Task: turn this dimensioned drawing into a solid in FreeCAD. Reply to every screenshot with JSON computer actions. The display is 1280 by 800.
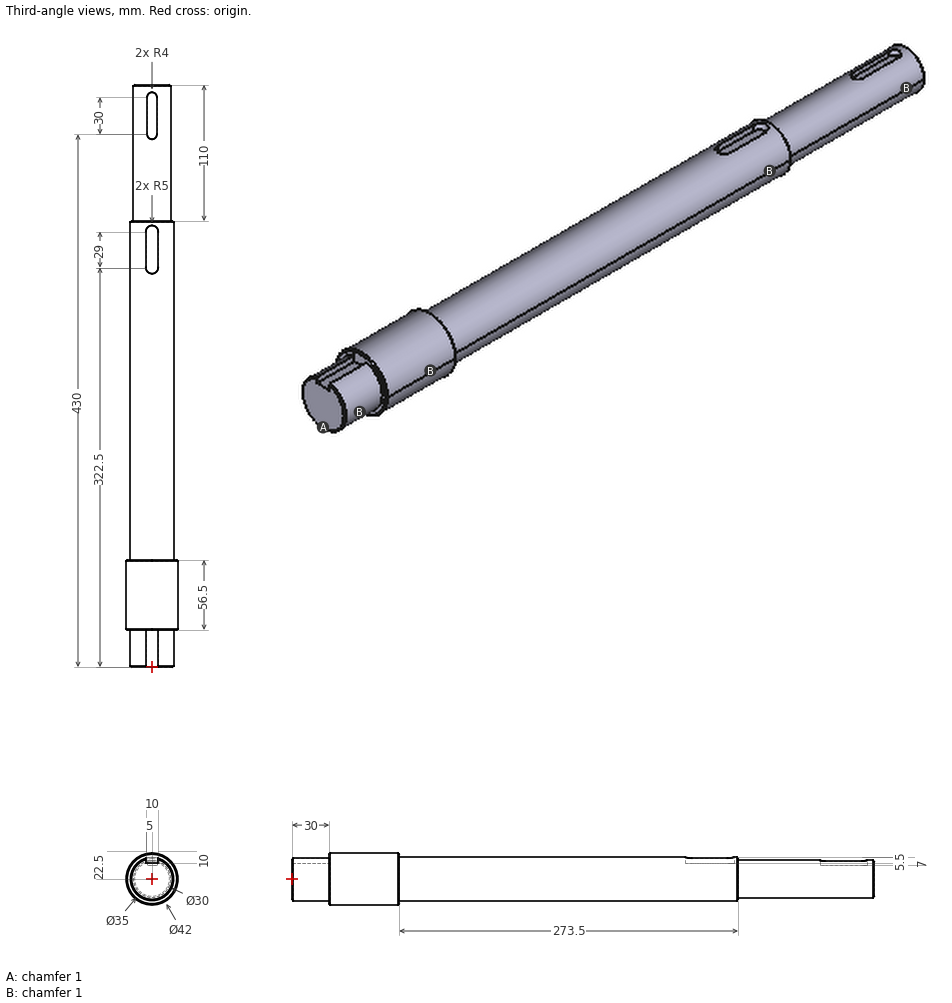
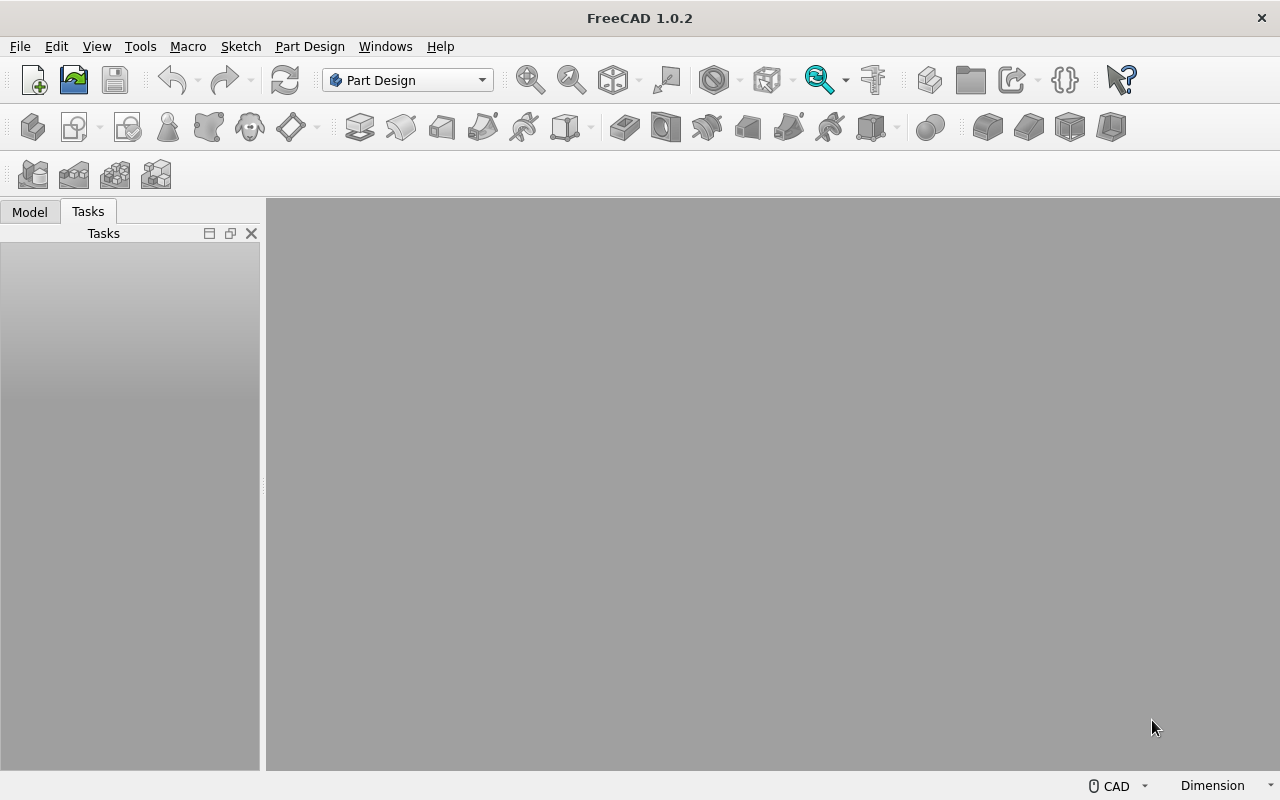
{"action": "key", "text": "ctrl+n"}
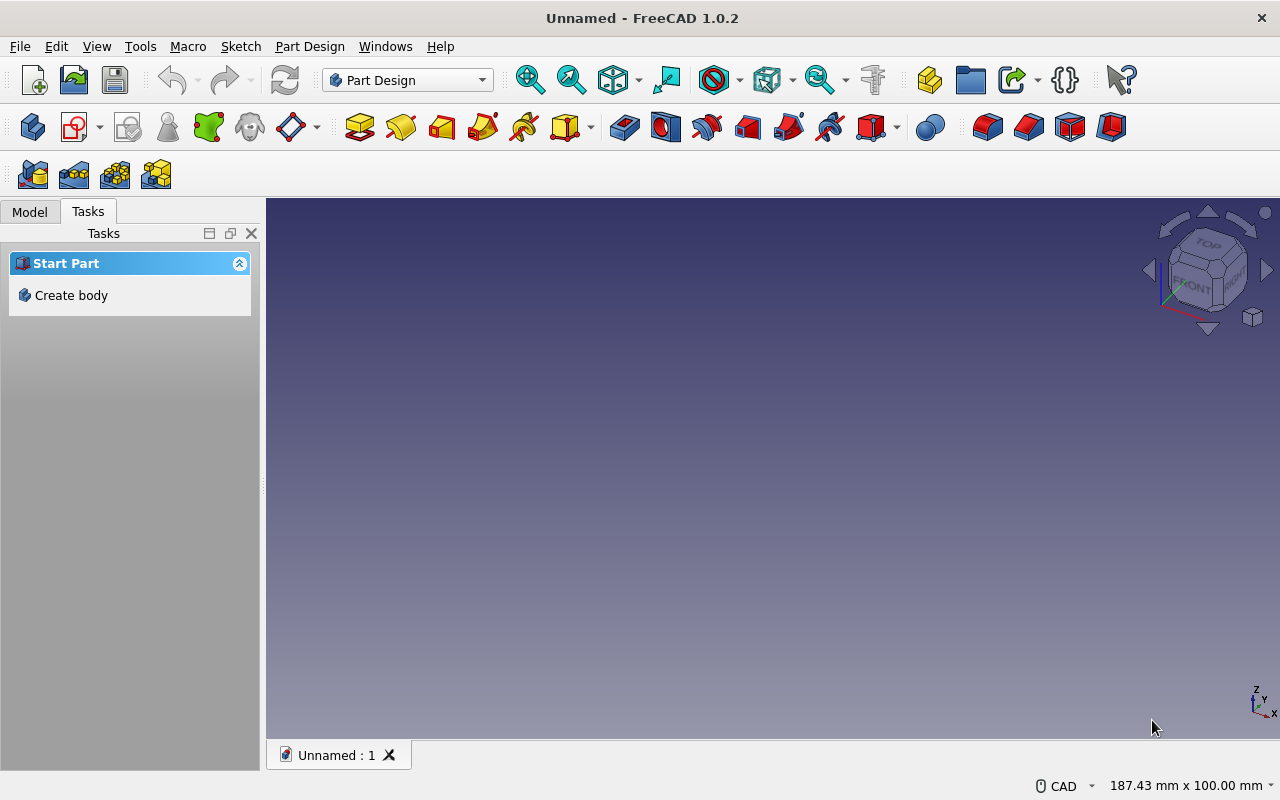
{"action": "left_click", "coordinate": [74, 128]}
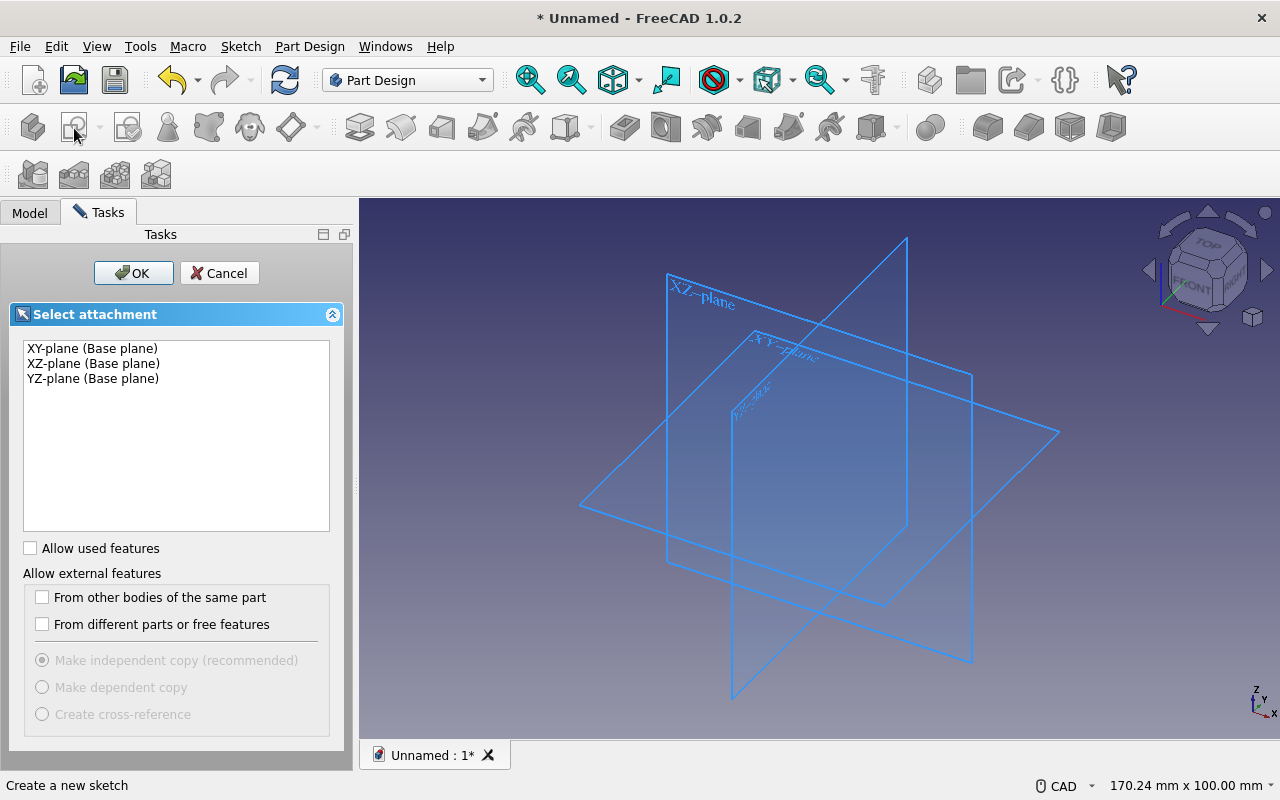
{"action": "left_click", "coordinate": [84, 364]}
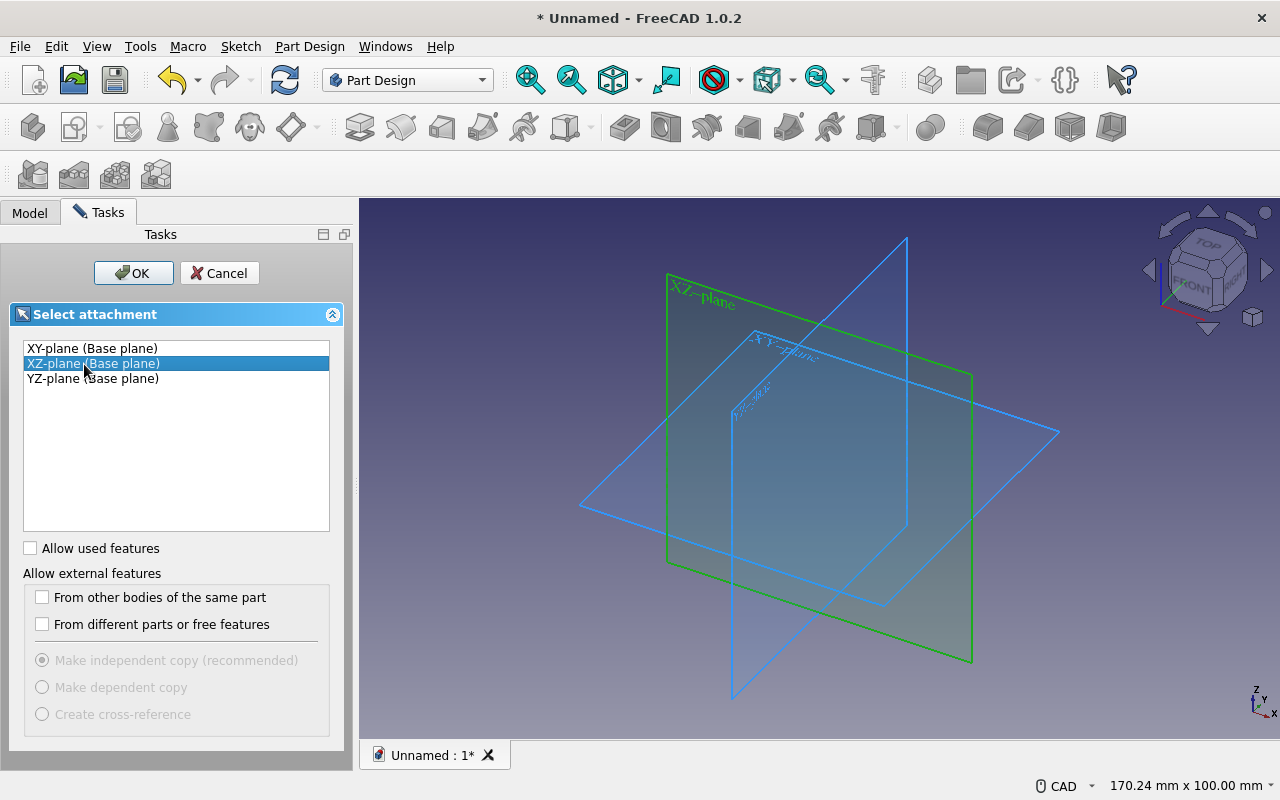
{"action": "left_click", "coordinate": [134, 273]}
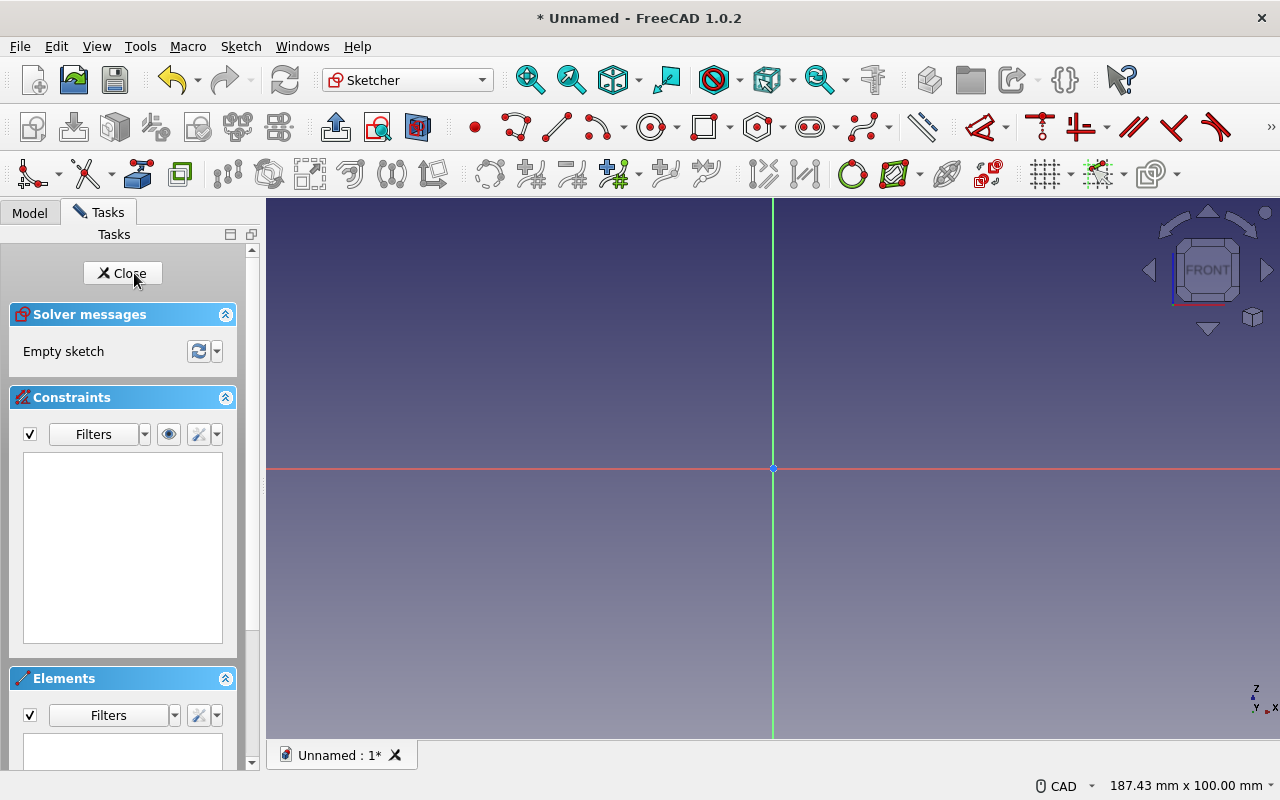
{"action": "scroll", "coordinate": [856, 468], "scroll_direction": "up", "scroll_amount": 3}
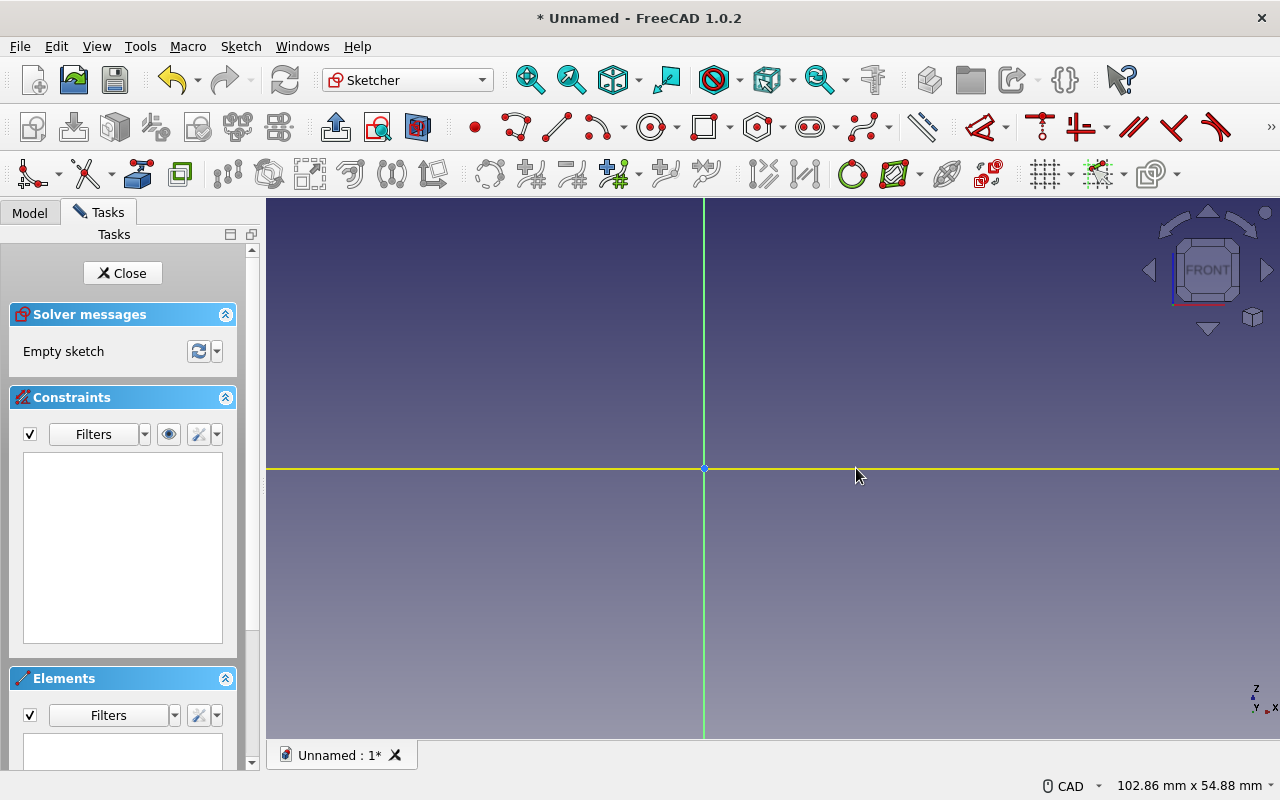
{"action": "left_click", "coordinate": [650, 128]}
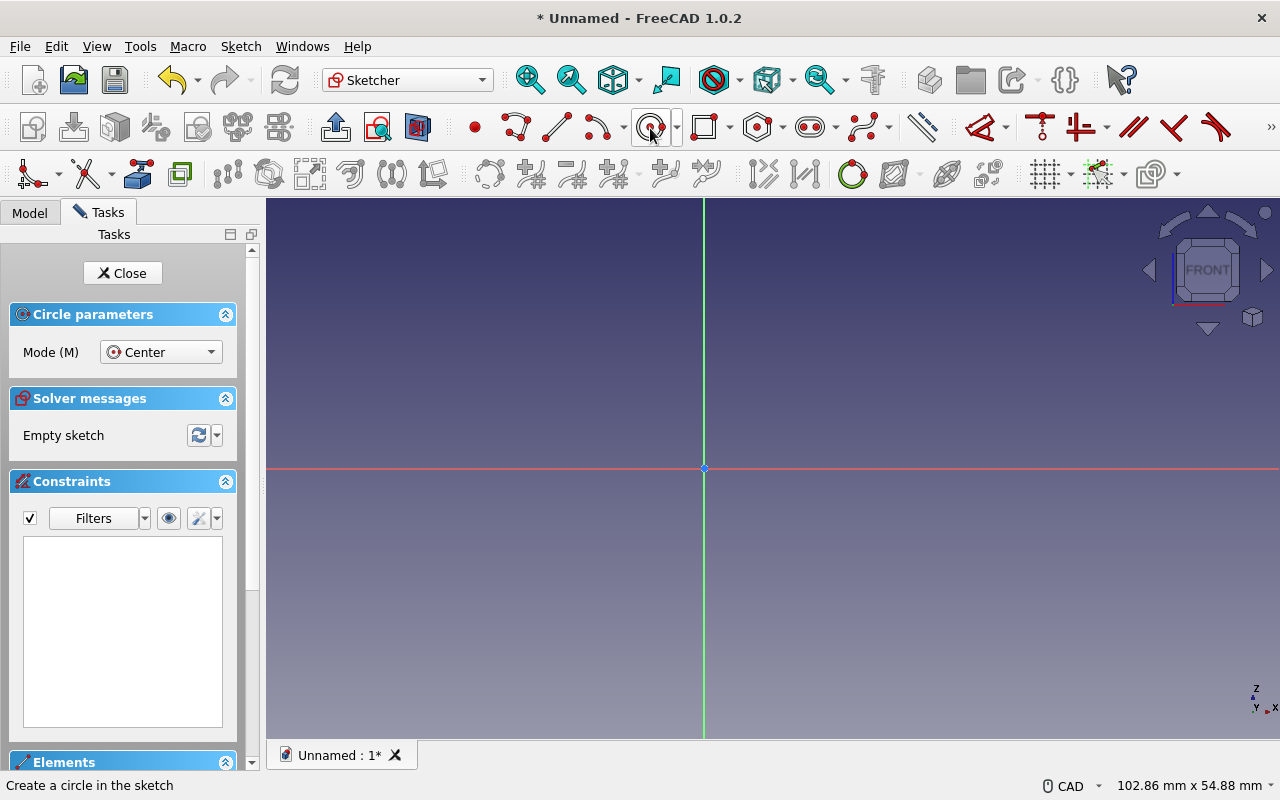
{"action": "left_click", "coordinate": [704, 468]}
{"action": "mouse_move", "coordinate": [826, 347]}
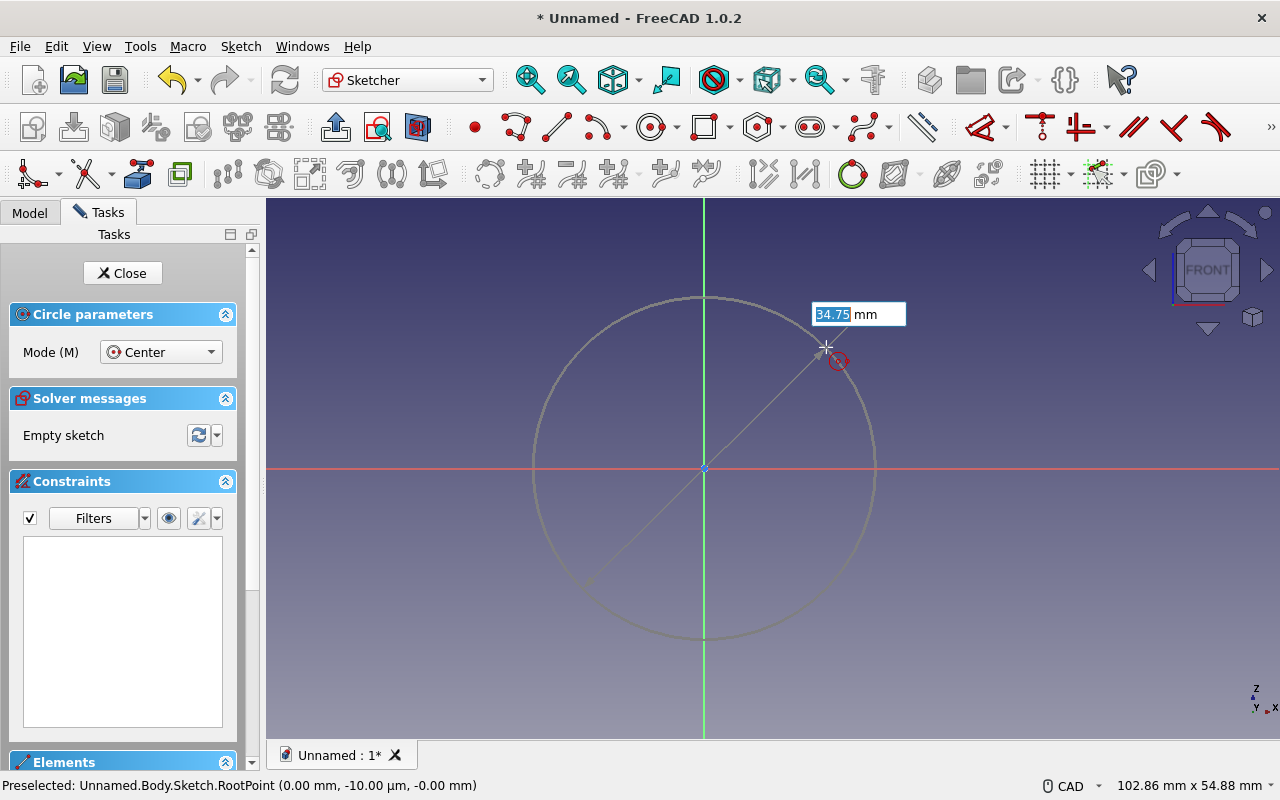
{"action": "type", "text": "35"}
{"action": "key", "text": "Return"}
{"action": "key", "text": "Escape"}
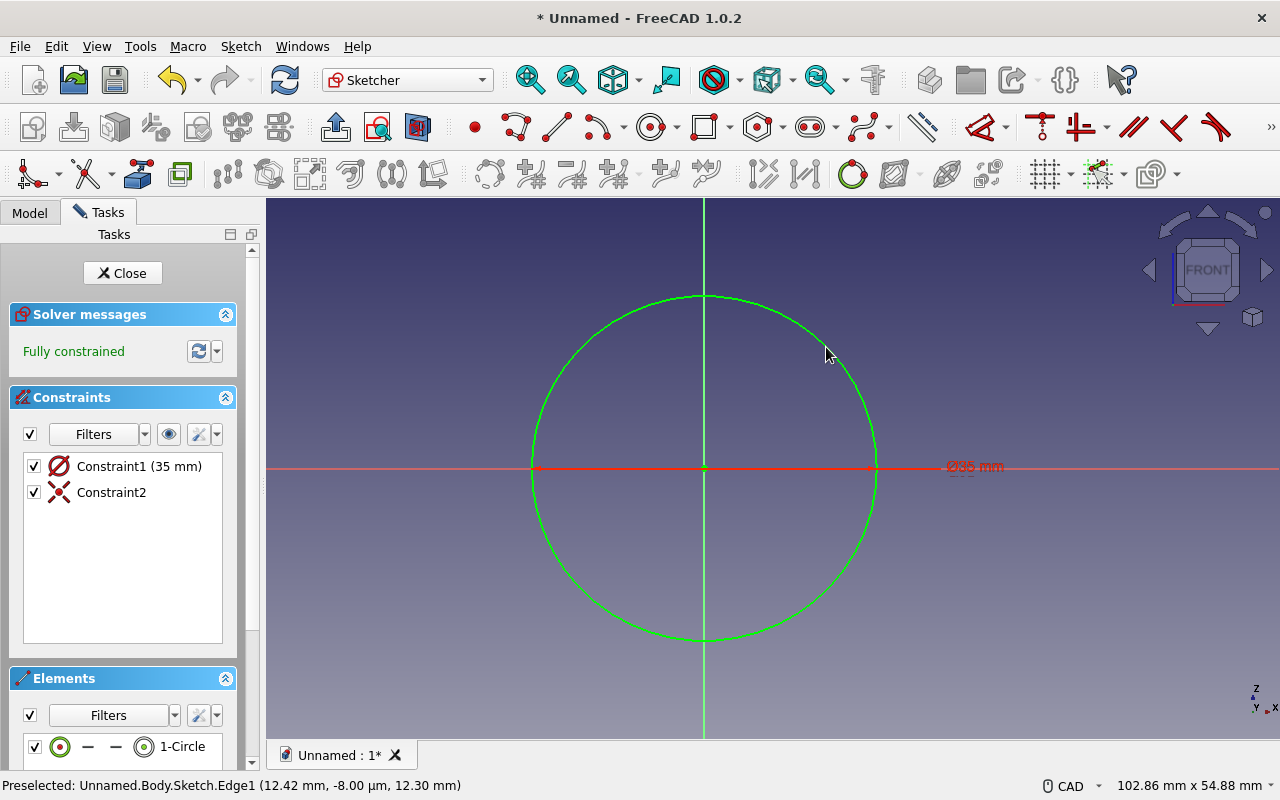
{"action": "left_click", "coordinate": [123, 273]}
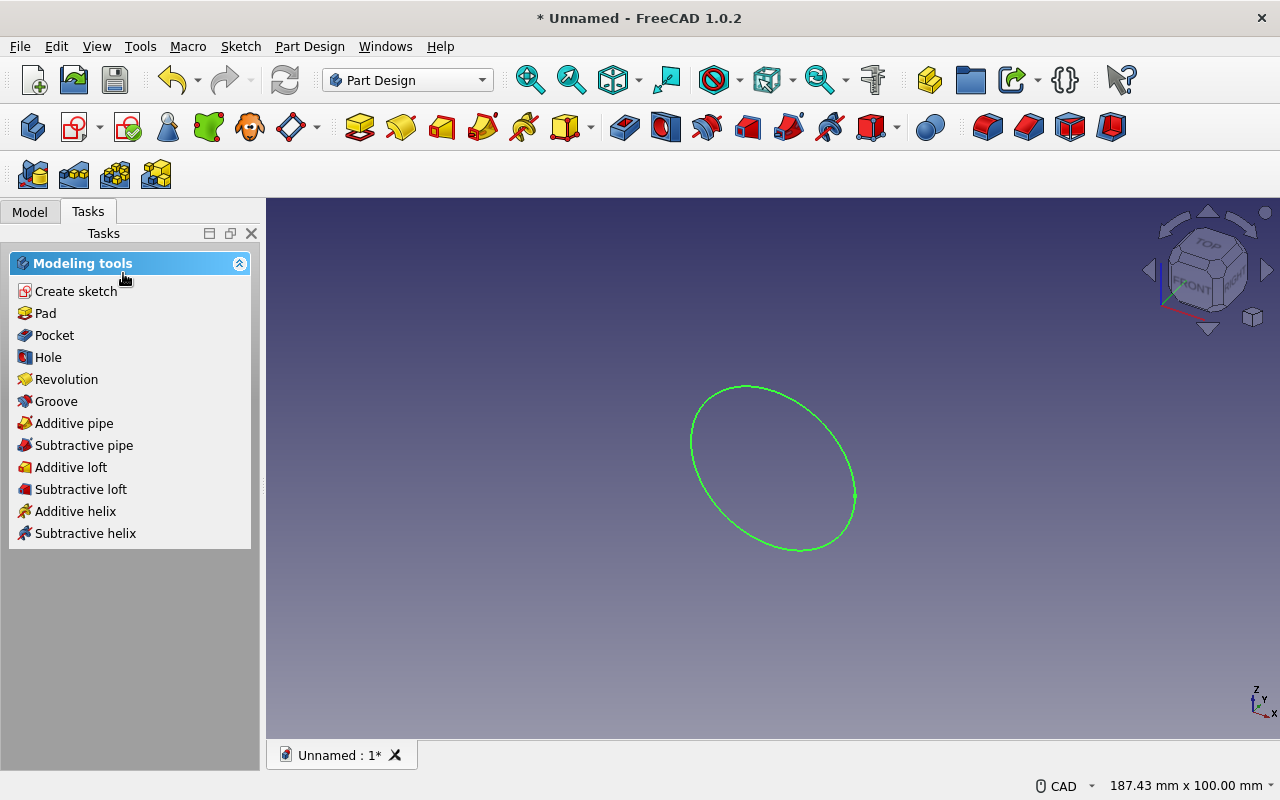
{"action": "left_click", "coordinate": [360, 128]}